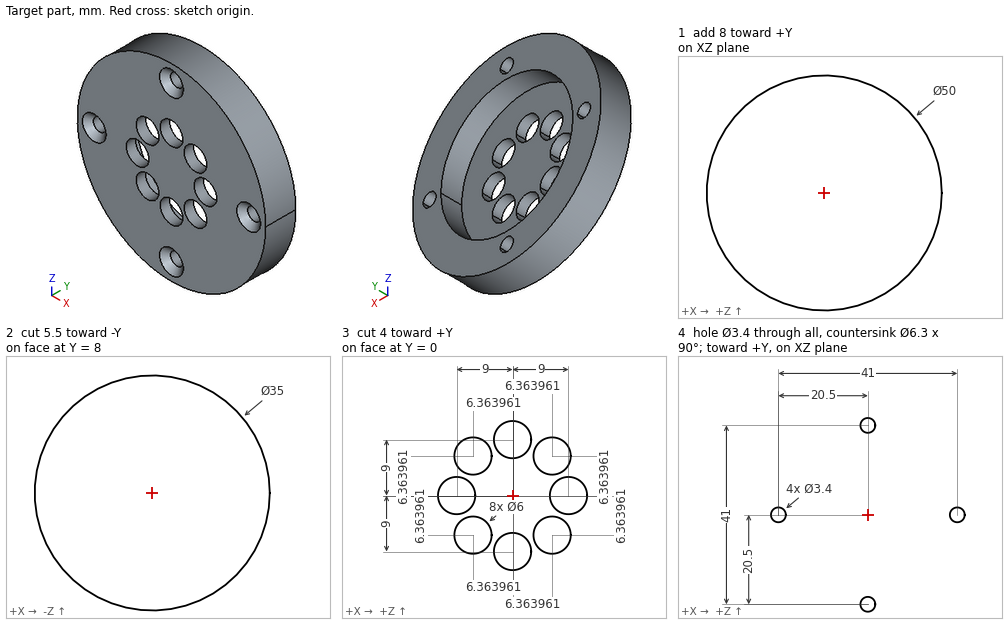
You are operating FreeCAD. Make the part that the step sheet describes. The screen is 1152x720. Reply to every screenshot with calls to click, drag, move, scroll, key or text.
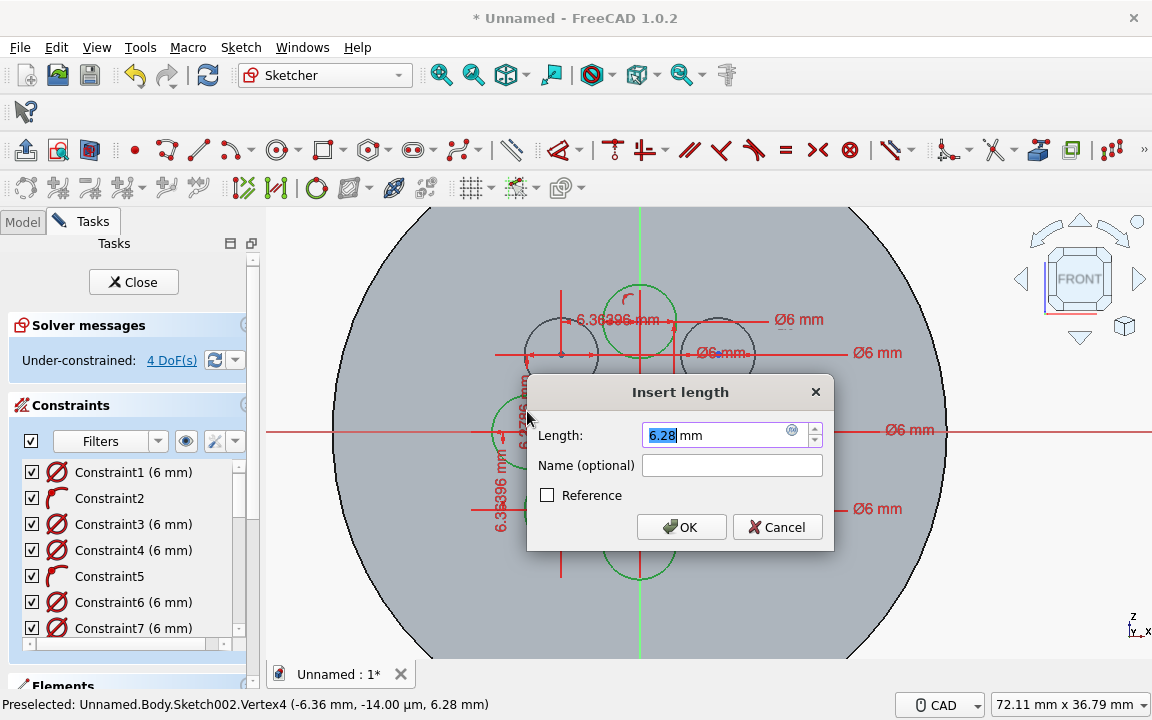
text(6.363961)
key(Return)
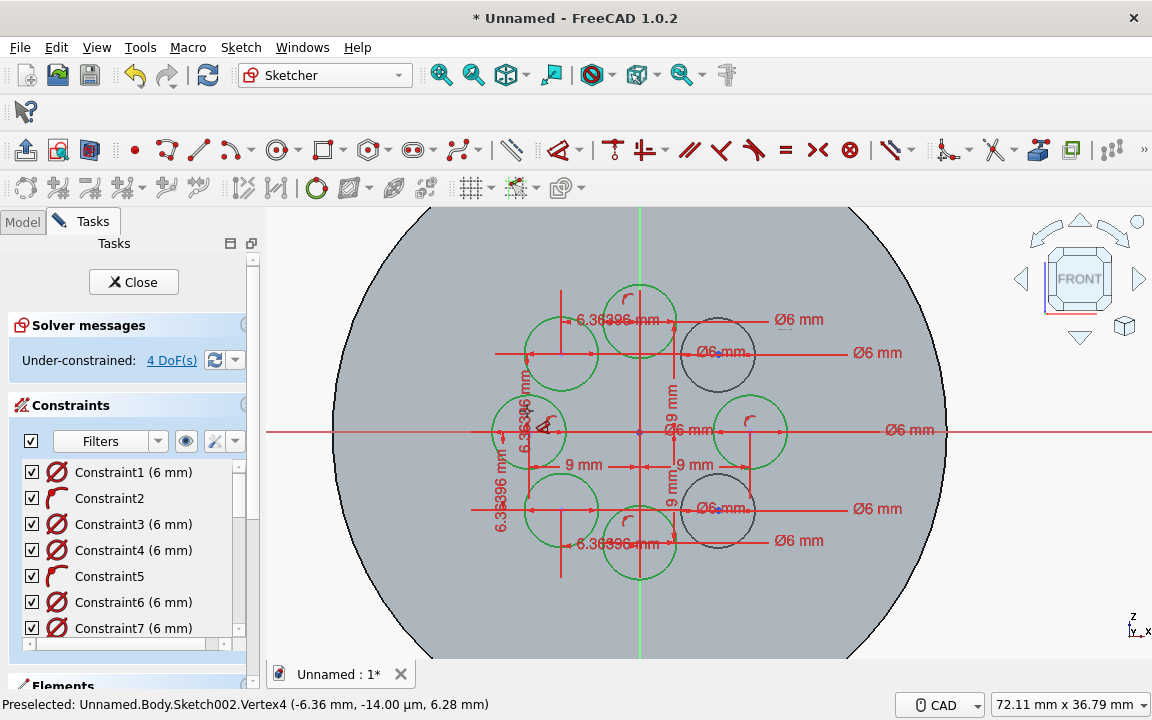
click(718, 355)
click(697, 297)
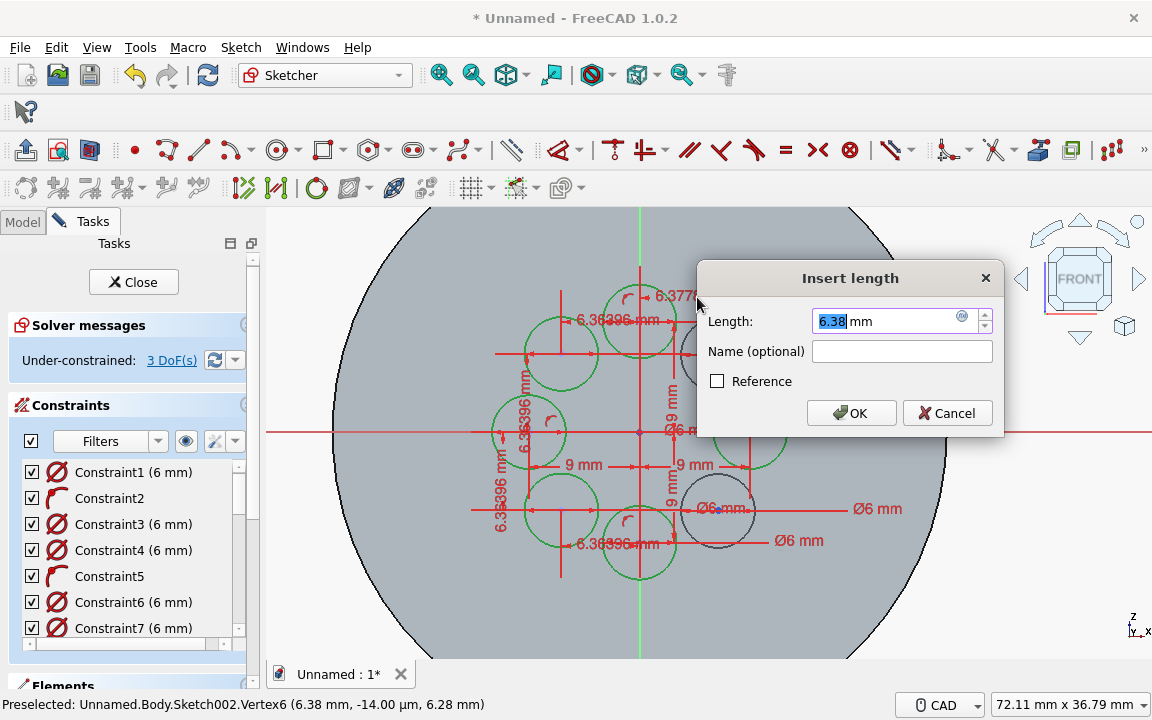
text(6.363961)
key(Return)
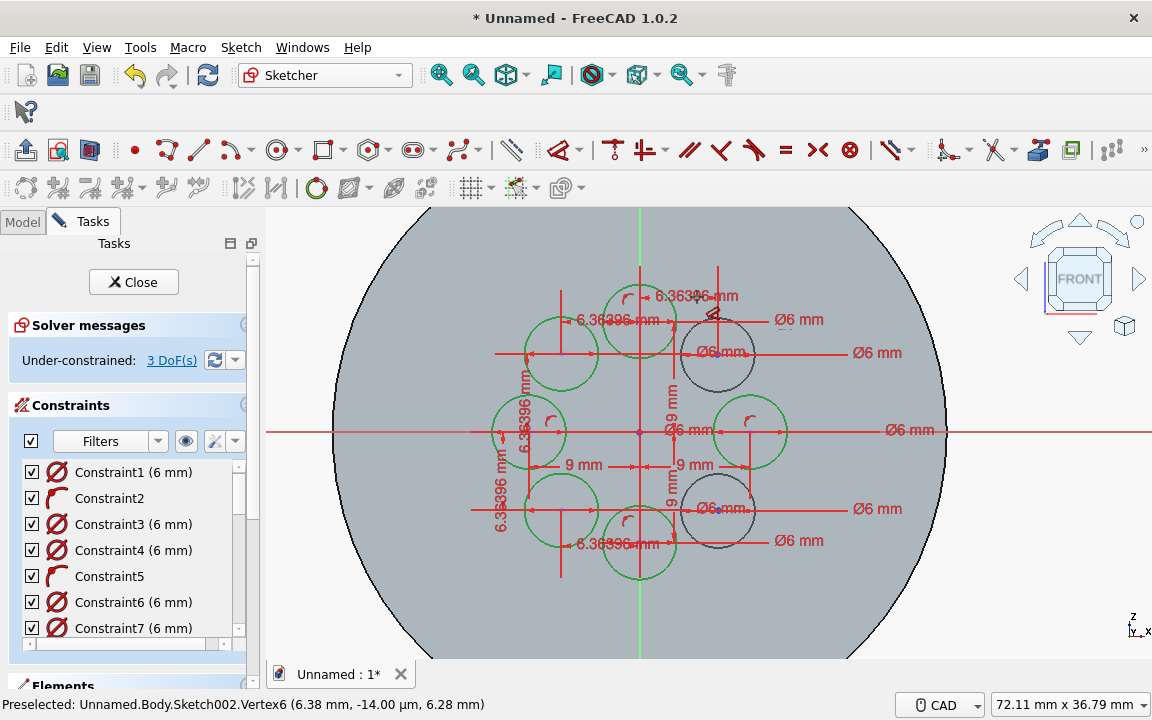
click(718, 355)
click(752, 411)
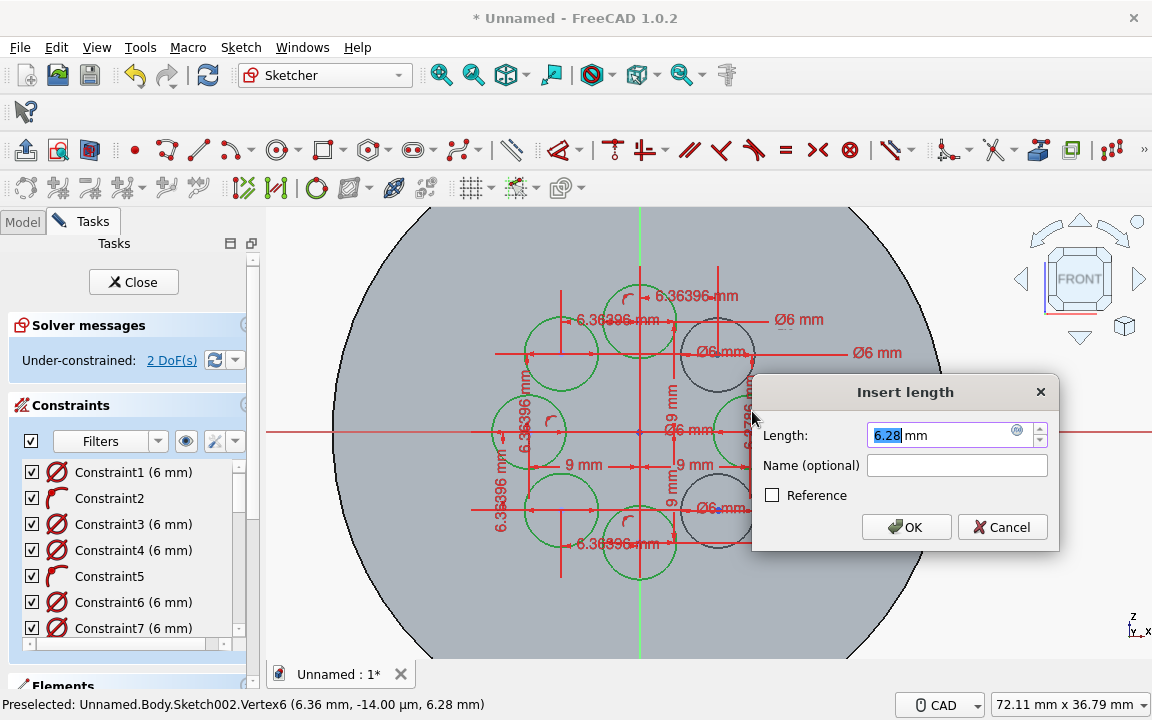
text(6.363961)
key(Return)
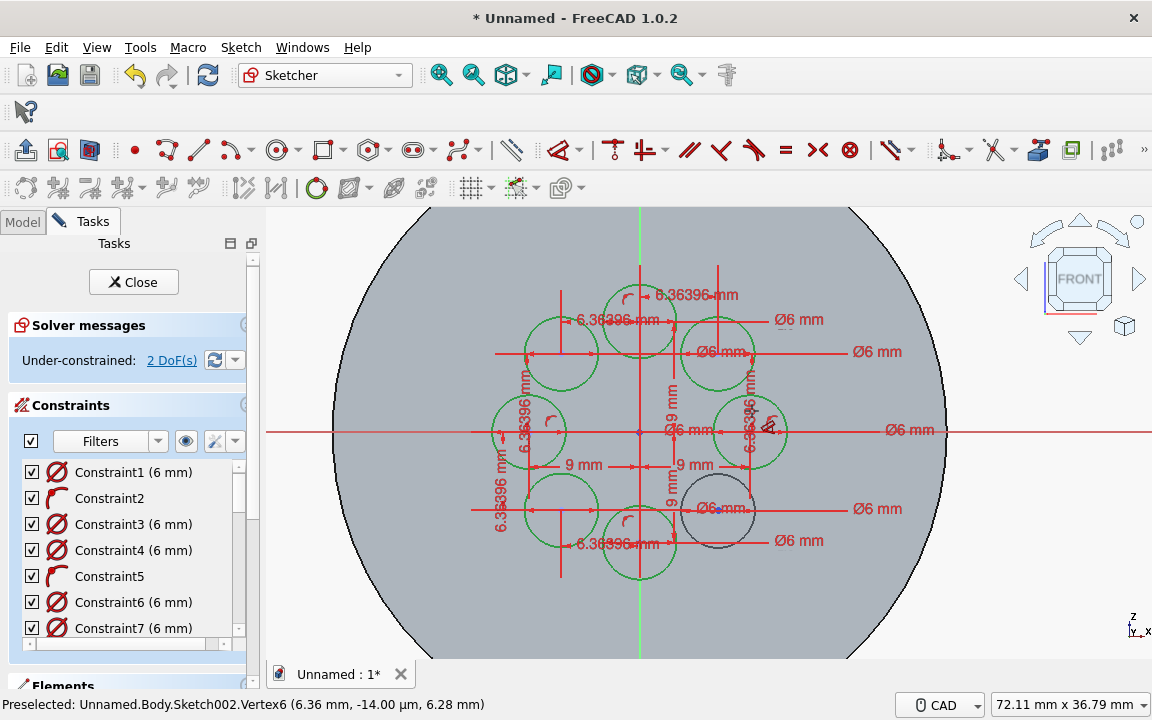
click(718, 511)
click(697, 569)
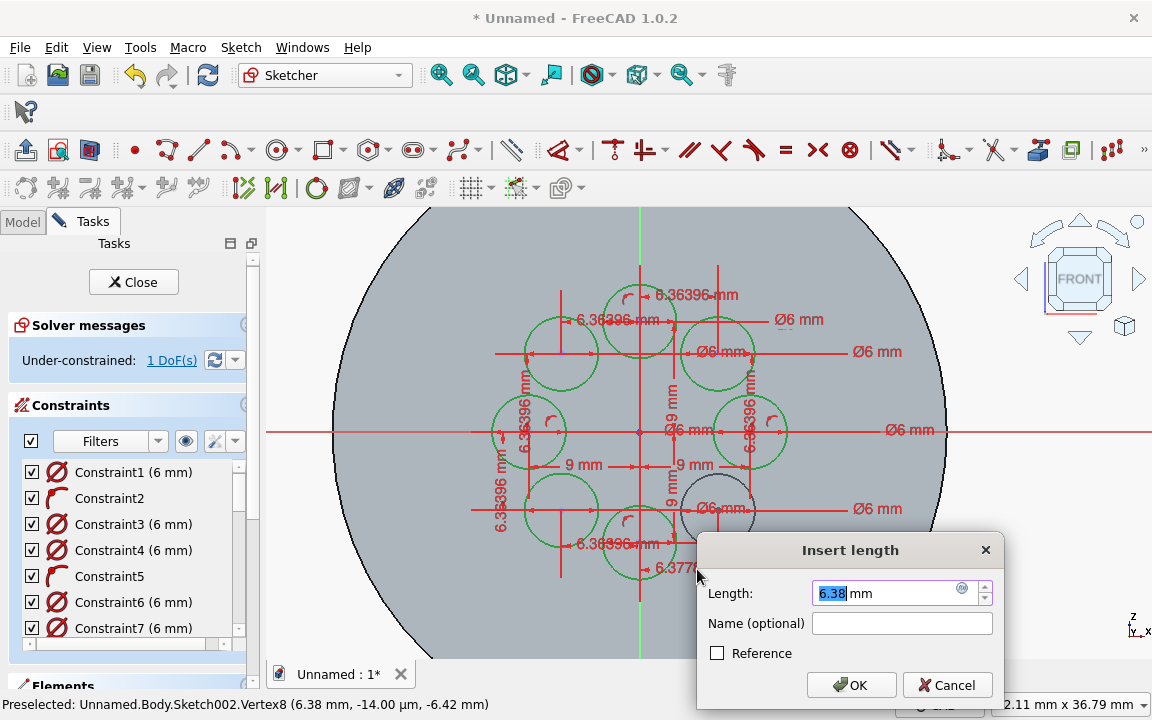
text(6.363961)
key(Return)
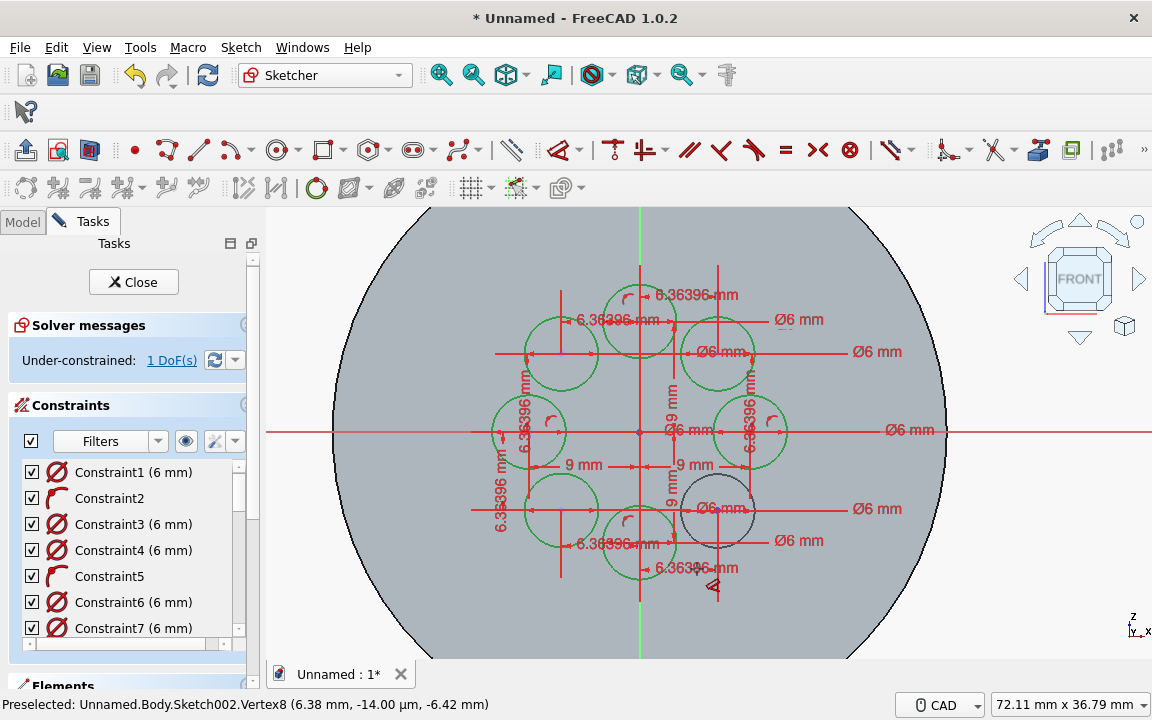
click(718, 511)
click(776, 490)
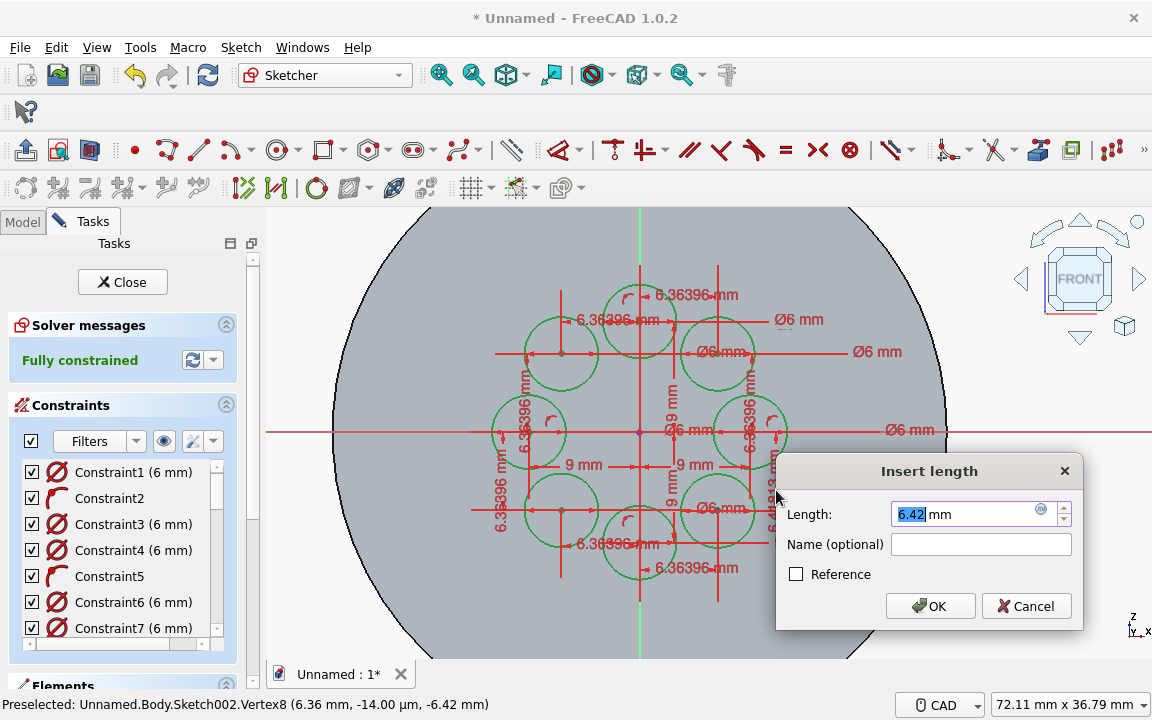
text(6.363961)
key(Return)
key(Escape)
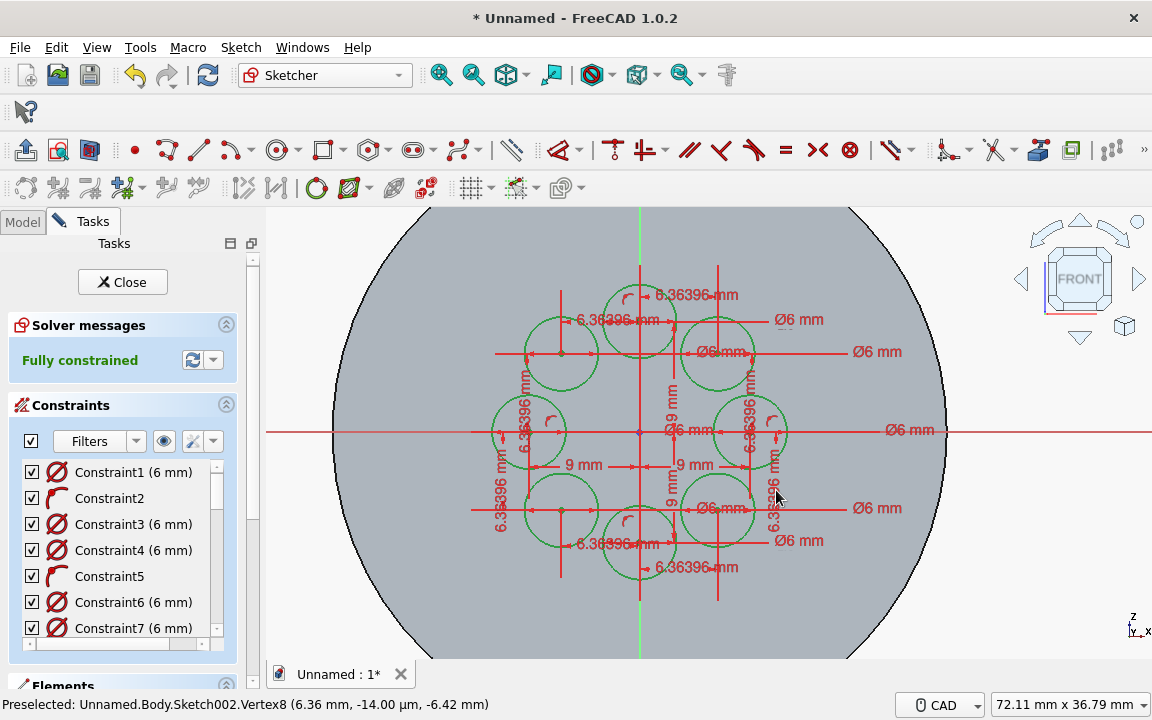
click(123, 282)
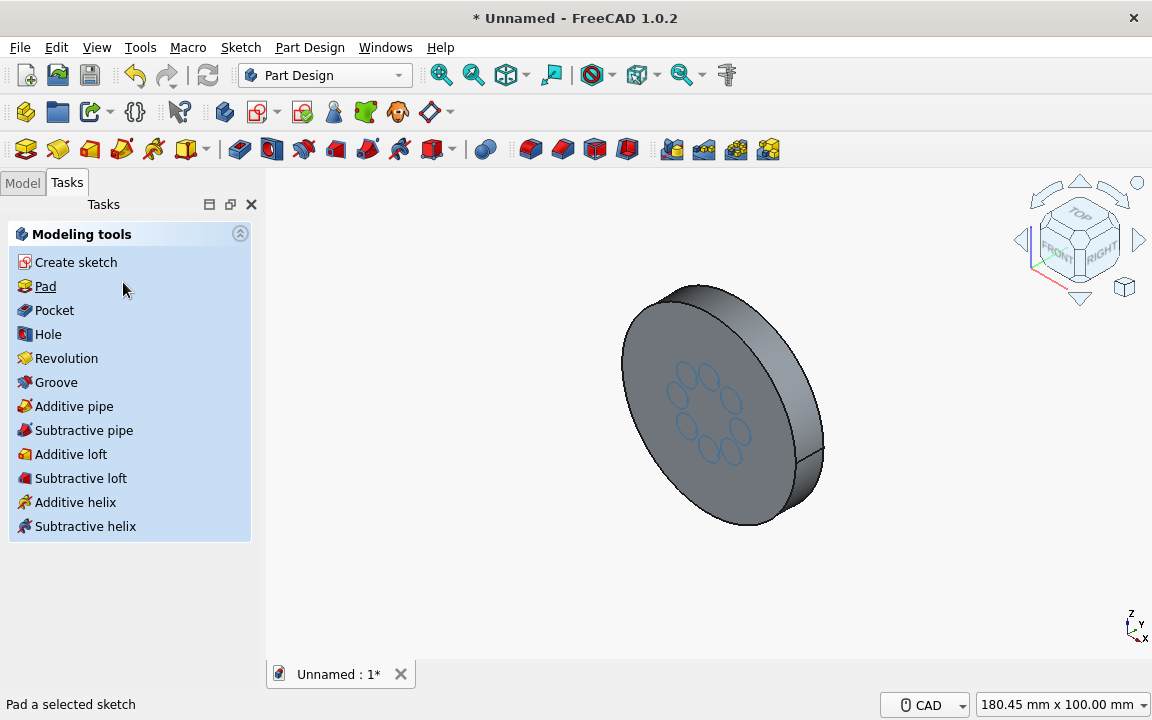
click(240, 150)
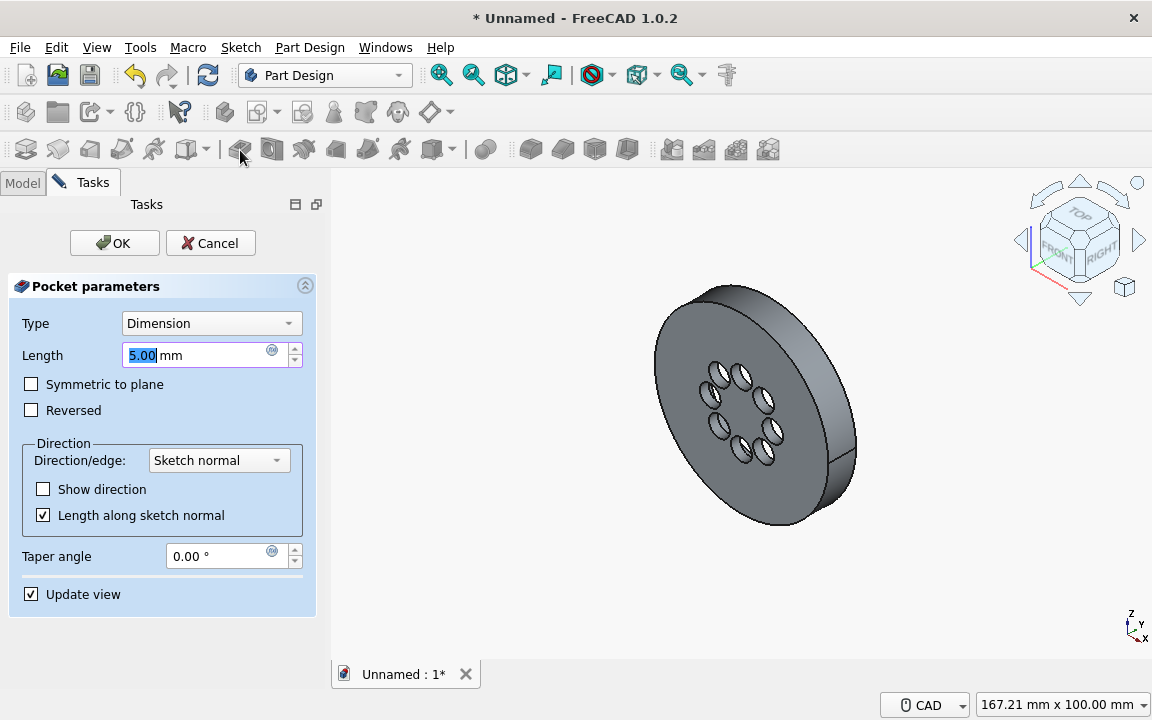
text(4)
key(Tab)